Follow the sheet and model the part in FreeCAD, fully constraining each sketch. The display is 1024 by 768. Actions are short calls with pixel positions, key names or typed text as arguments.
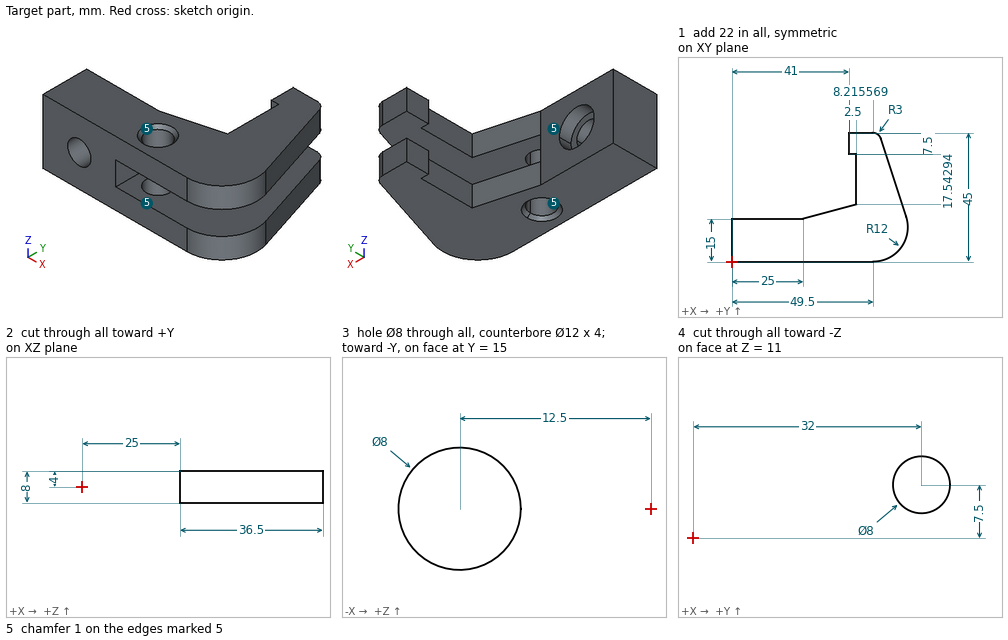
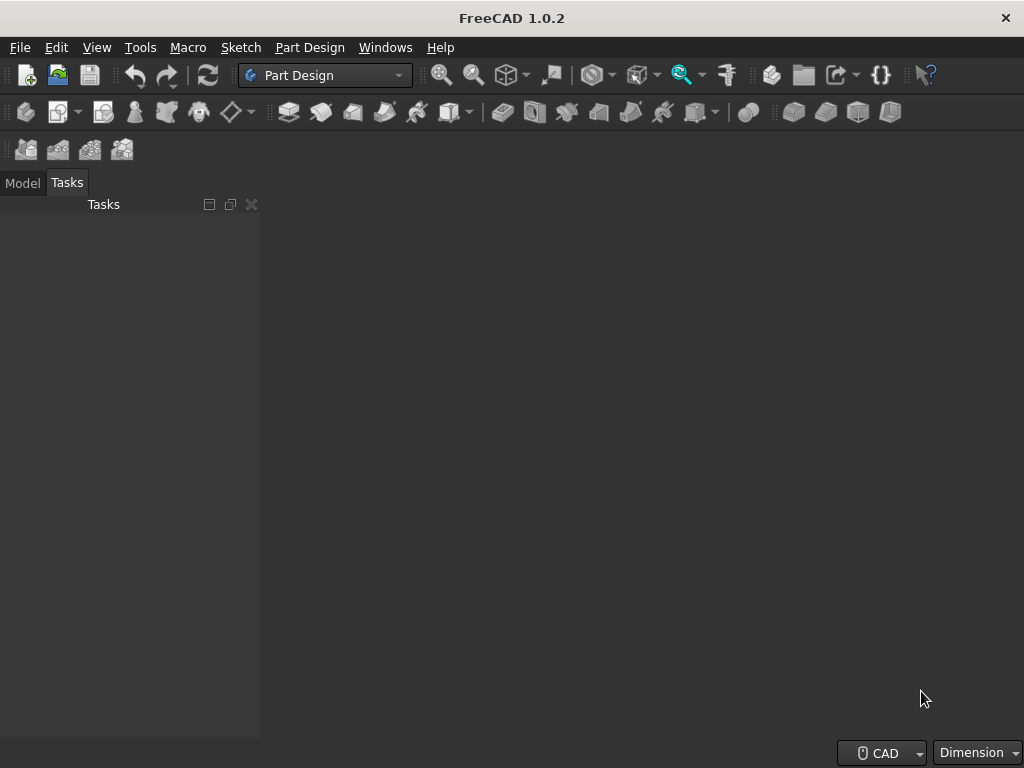
click(26, 76)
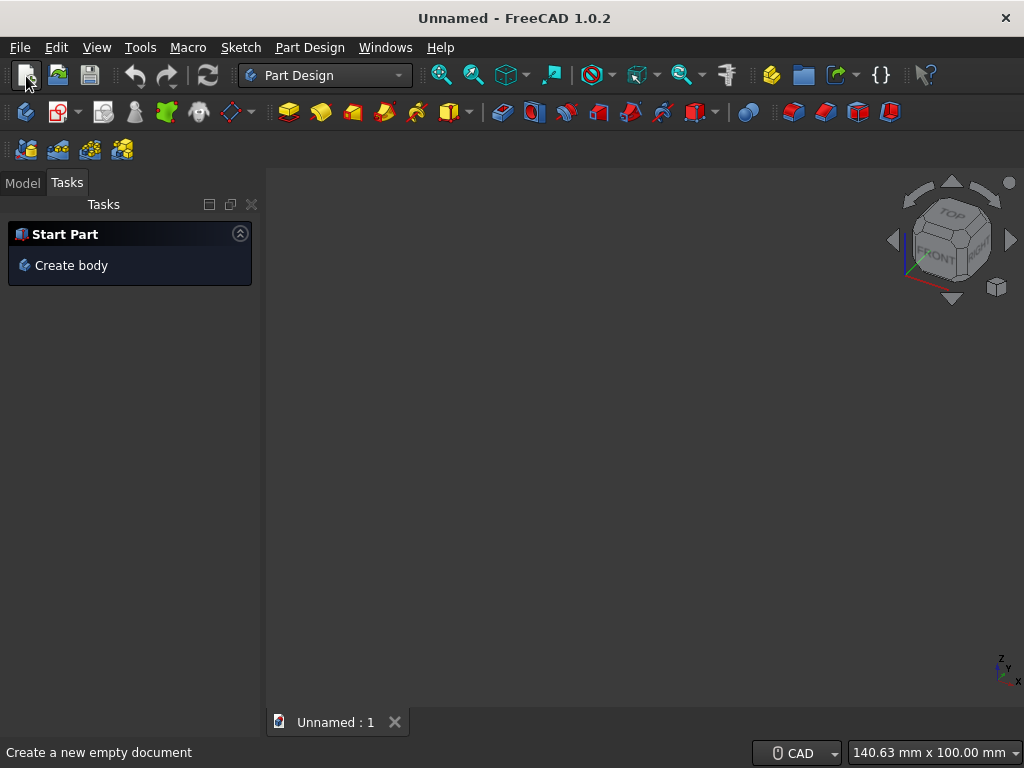
click(58, 112)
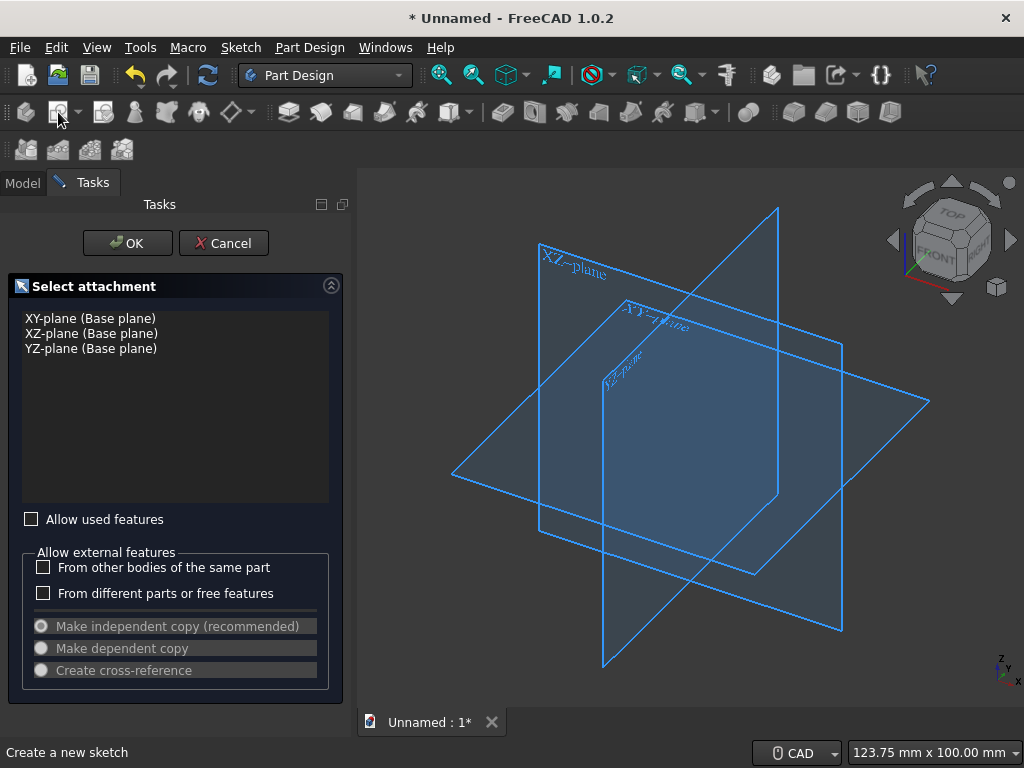
click(82, 318)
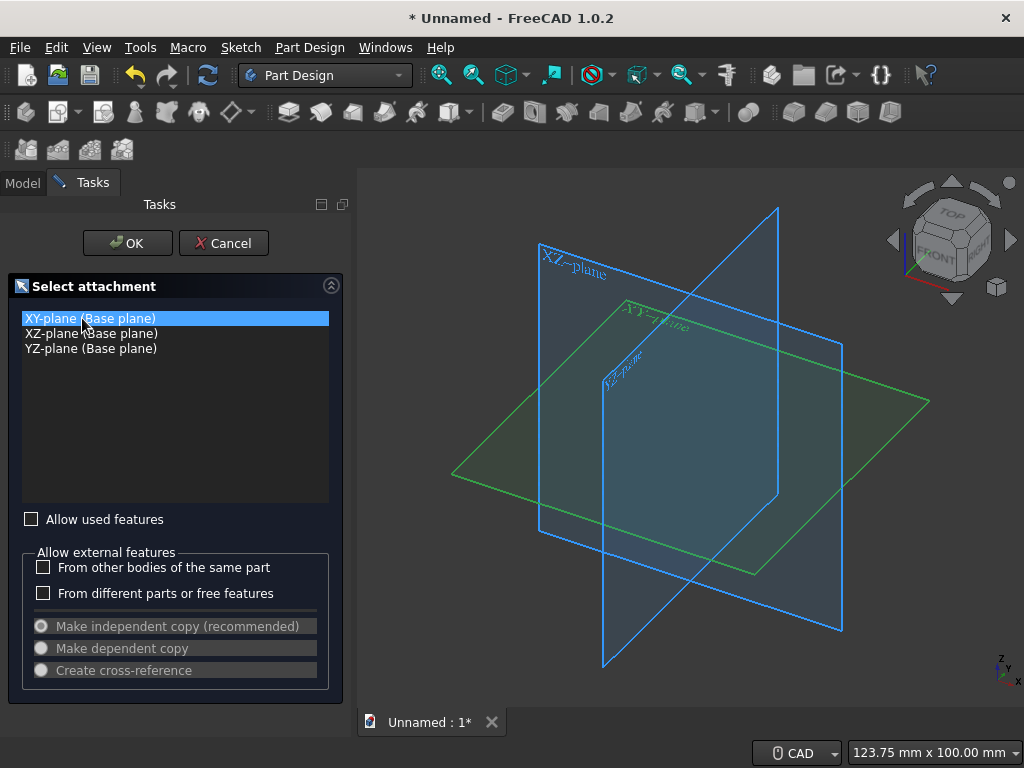
click(128, 243)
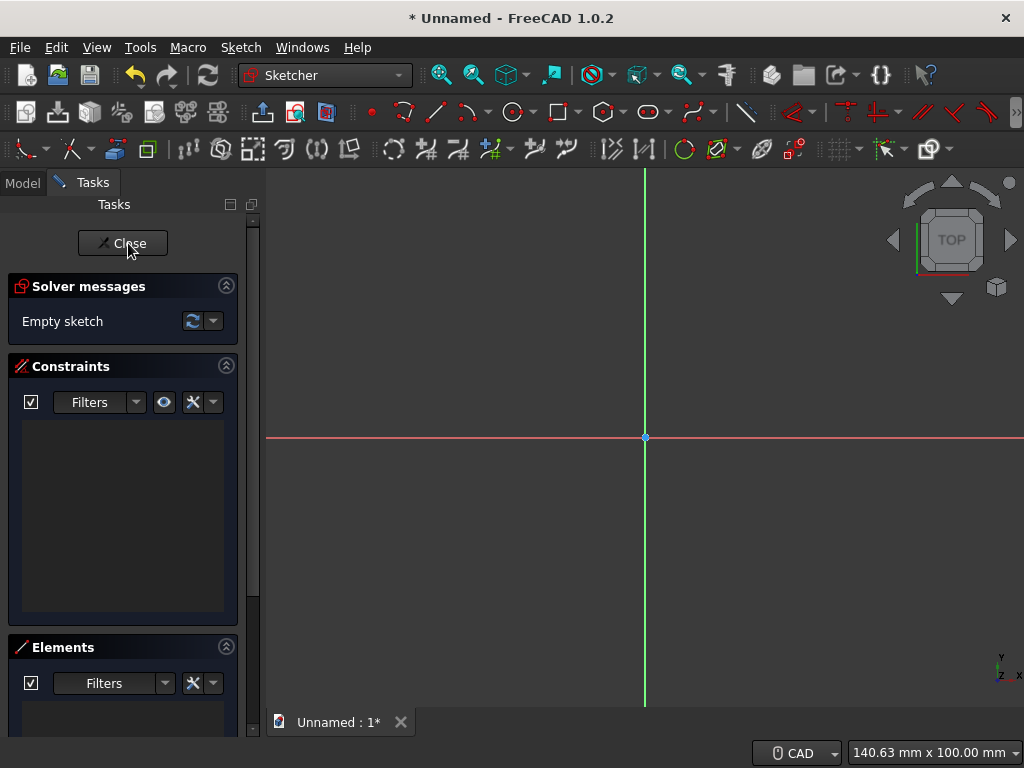
scroll(294, 679, down, 2)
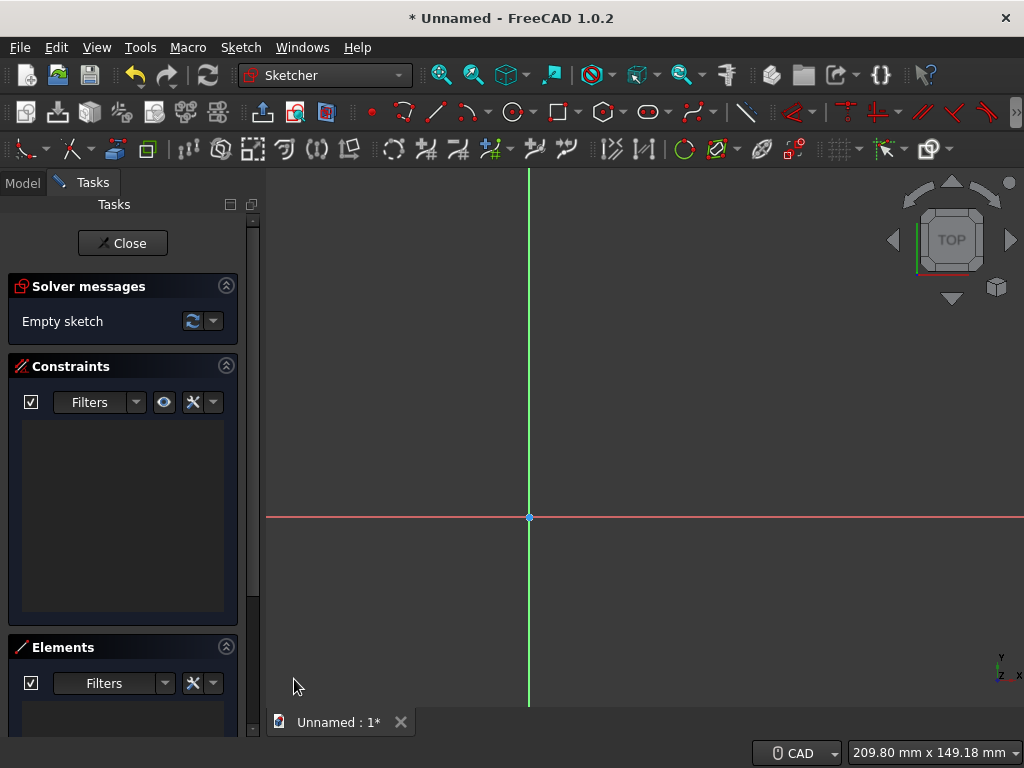
scroll(716, 434, up, 3)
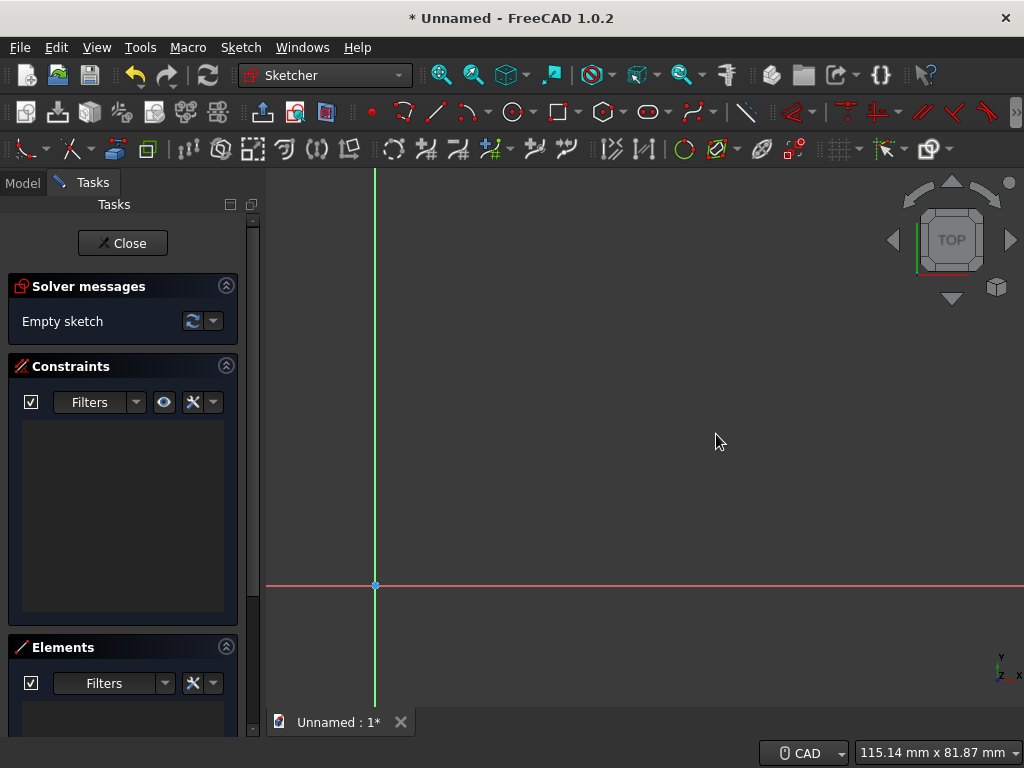
click(436, 112)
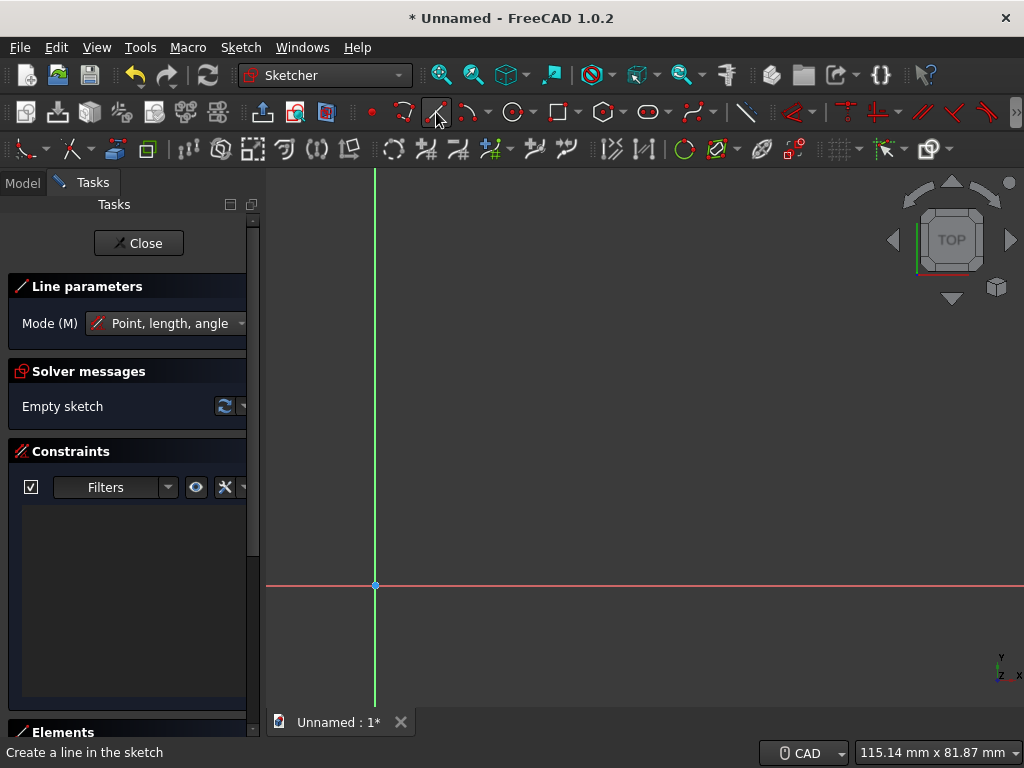
click(776, 482)
click(718, 303)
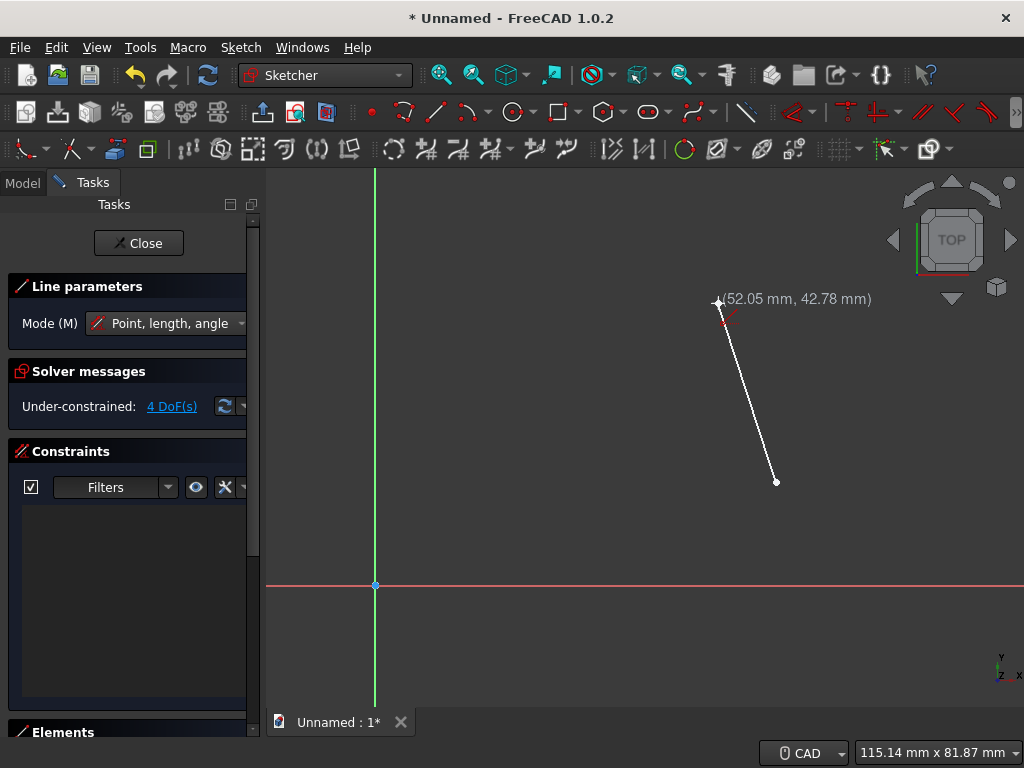
key(g)
key(m)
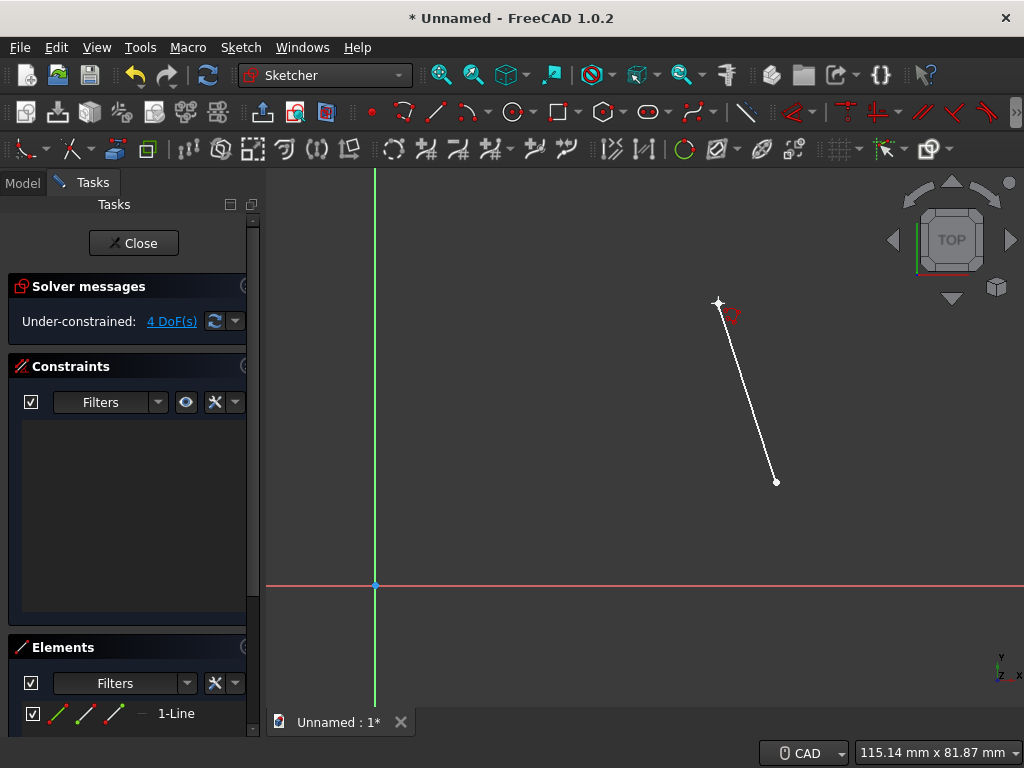
click(699, 289)
click(645, 289)
click(645, 339)
click(662, 339)
click(662, 454)
click(540, 487)
click(375, 487)
click(375, 586)
click(701, 577)
right_click(701, 577)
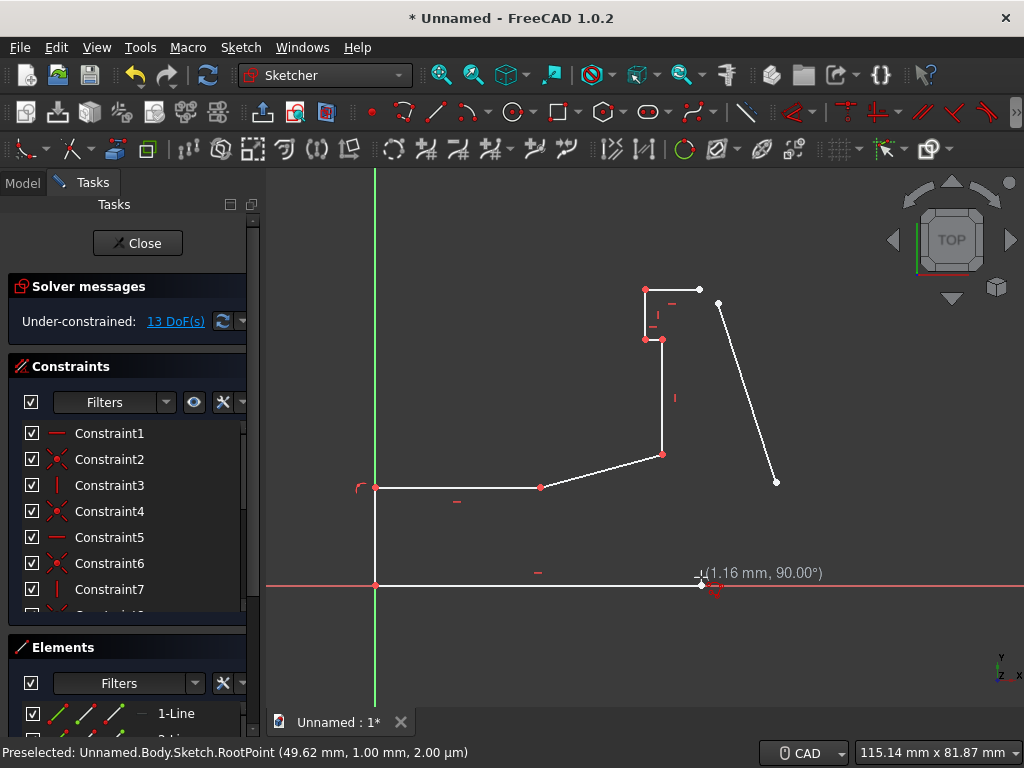
key(g)
key(3)
key(a)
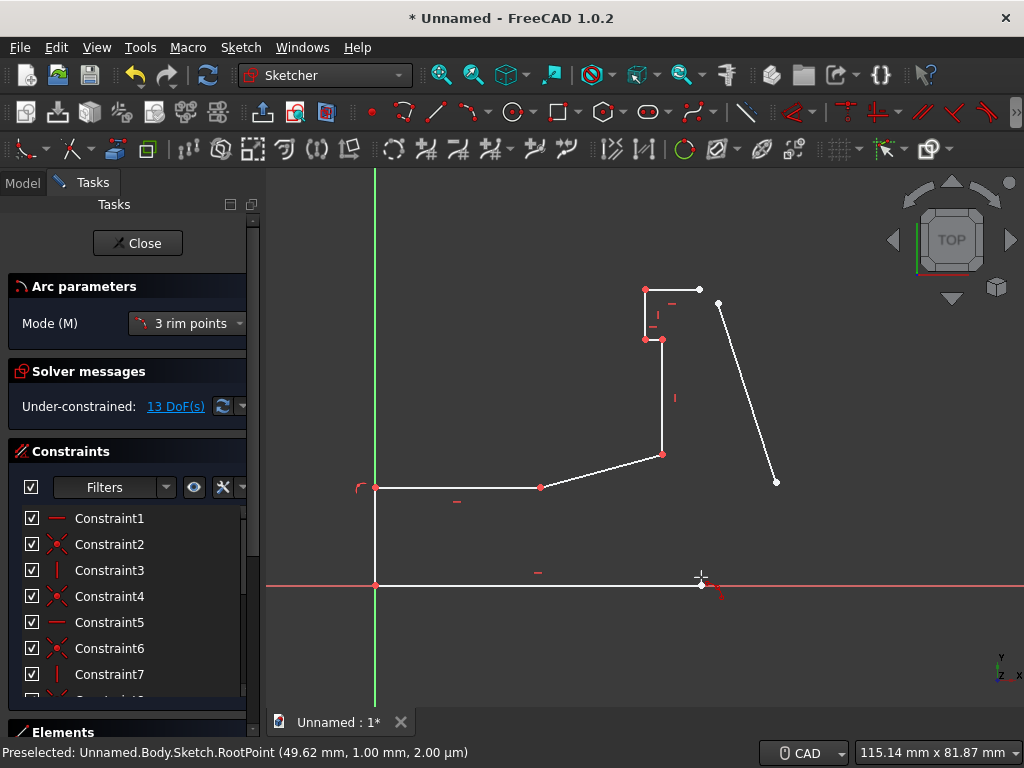
click(718, 304)
click(699, 290)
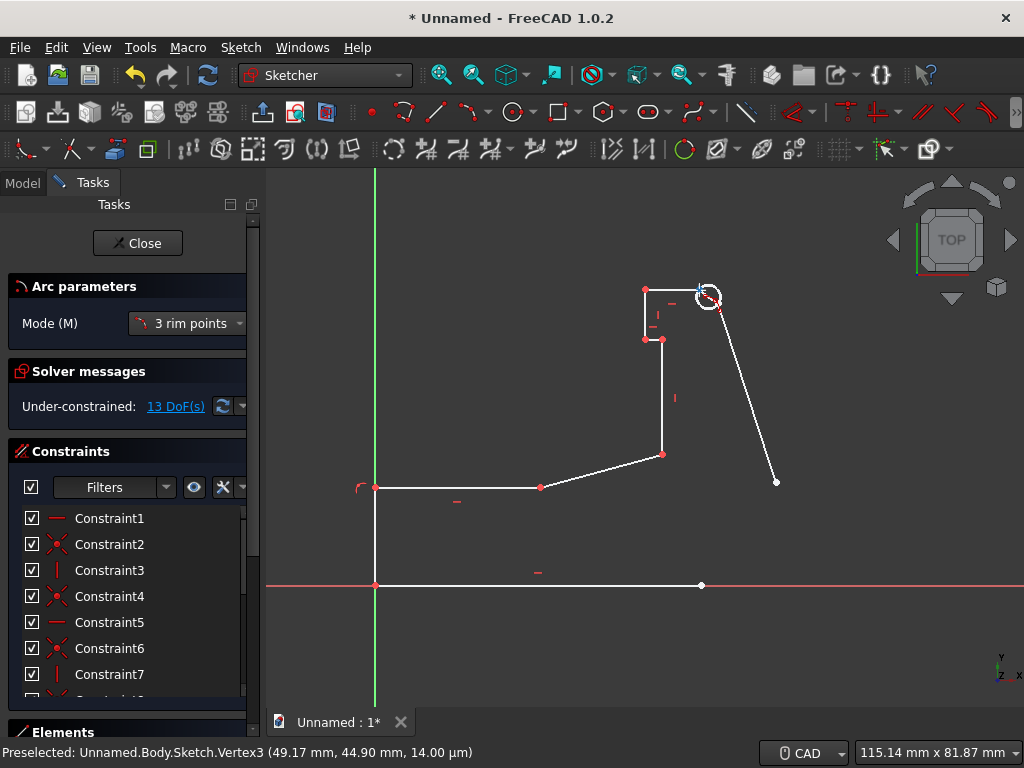
scroll(711, 293, up, 8)